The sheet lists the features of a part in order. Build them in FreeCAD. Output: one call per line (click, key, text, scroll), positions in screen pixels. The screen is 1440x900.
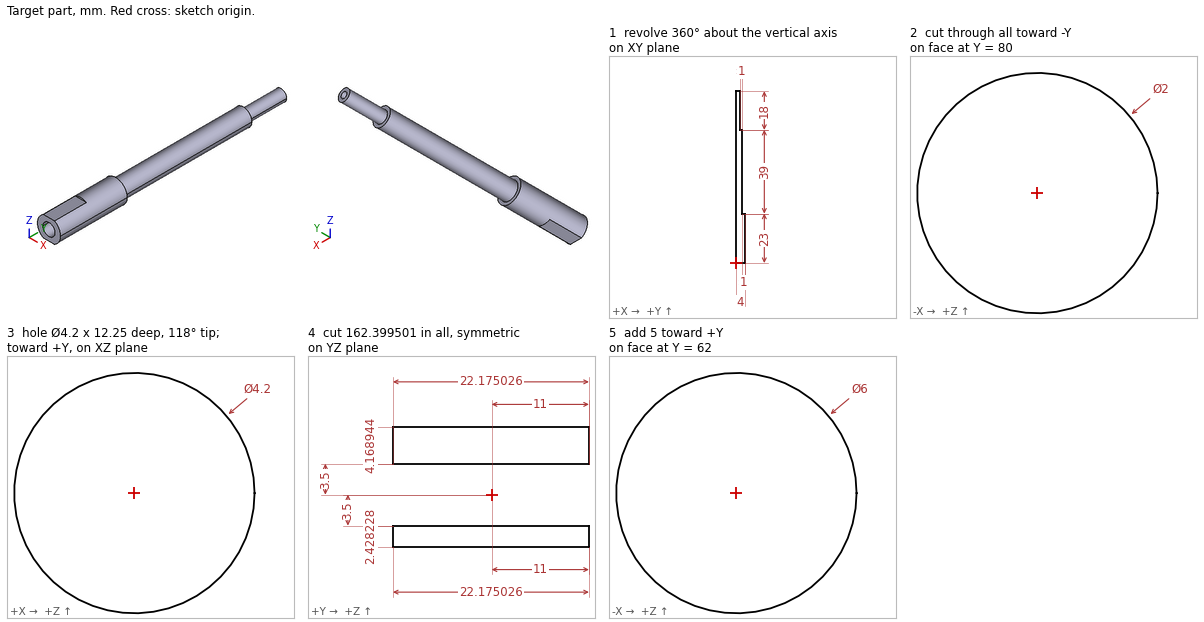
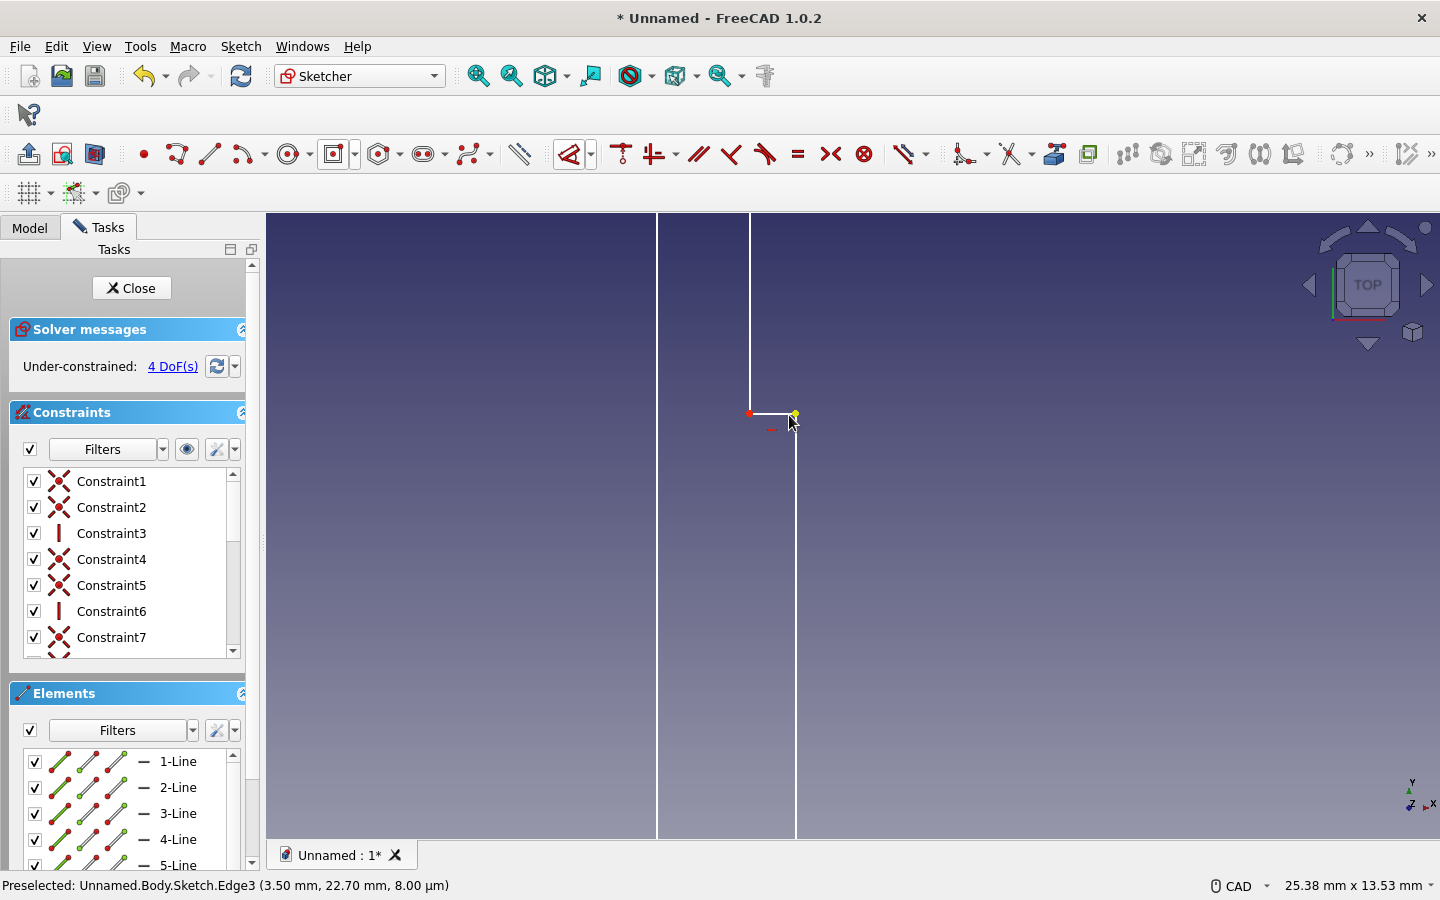
click(782, 414)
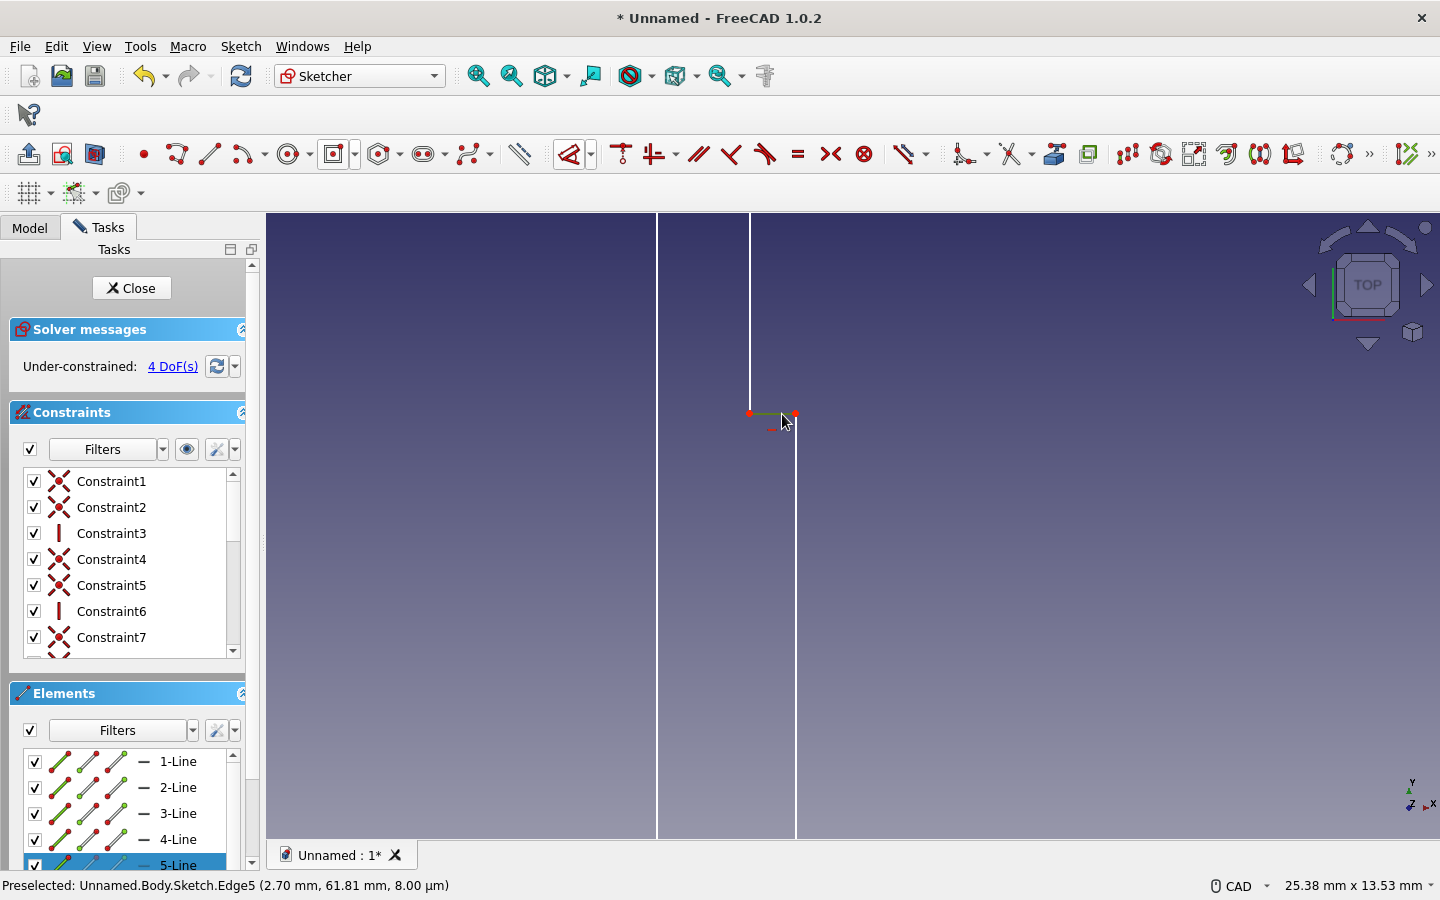
key(l)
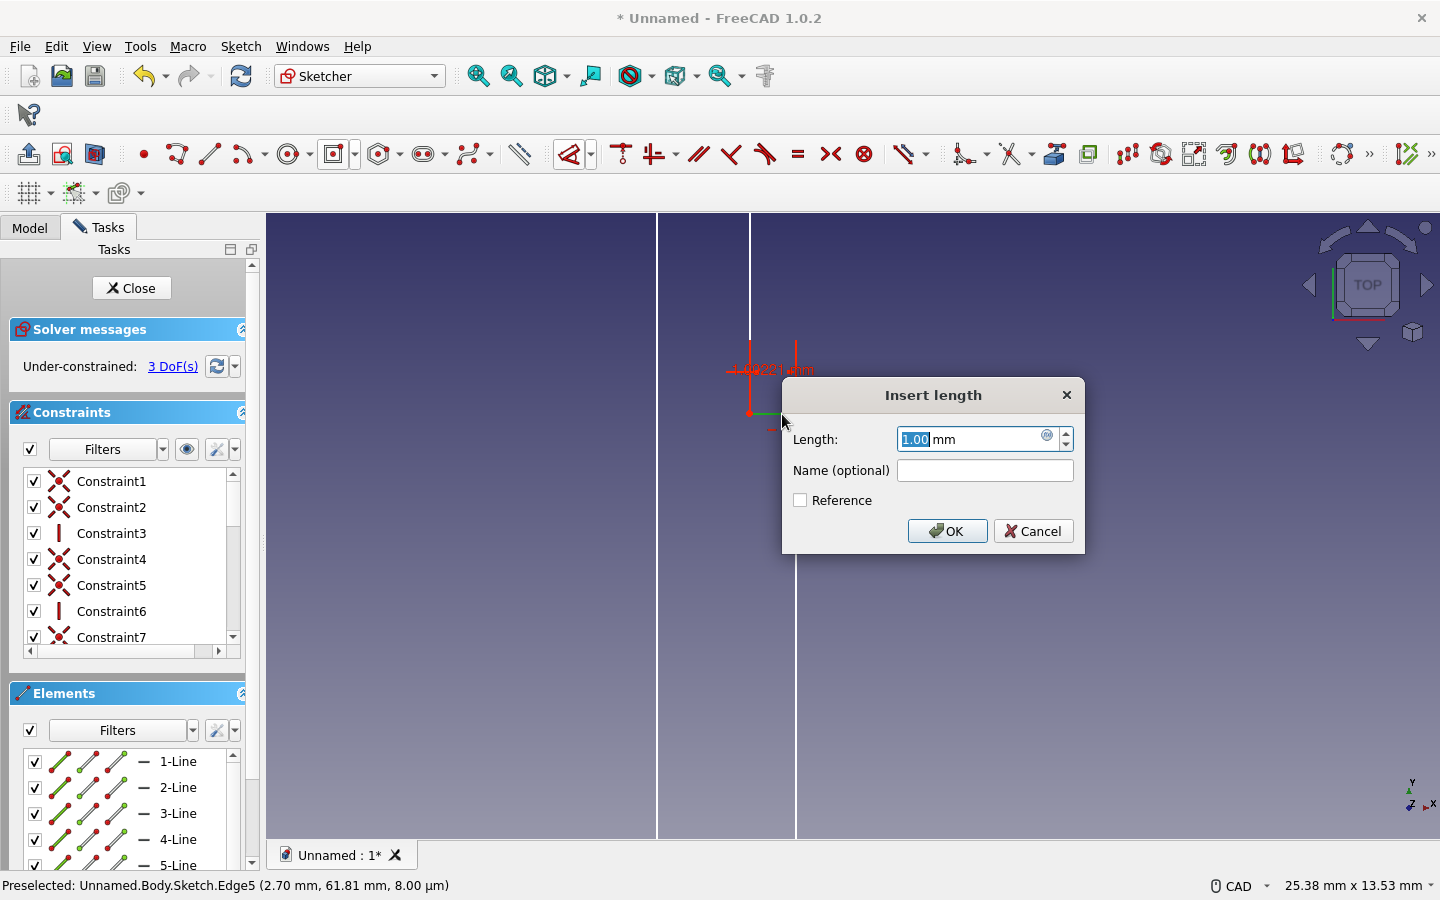
text(1)
key(Return)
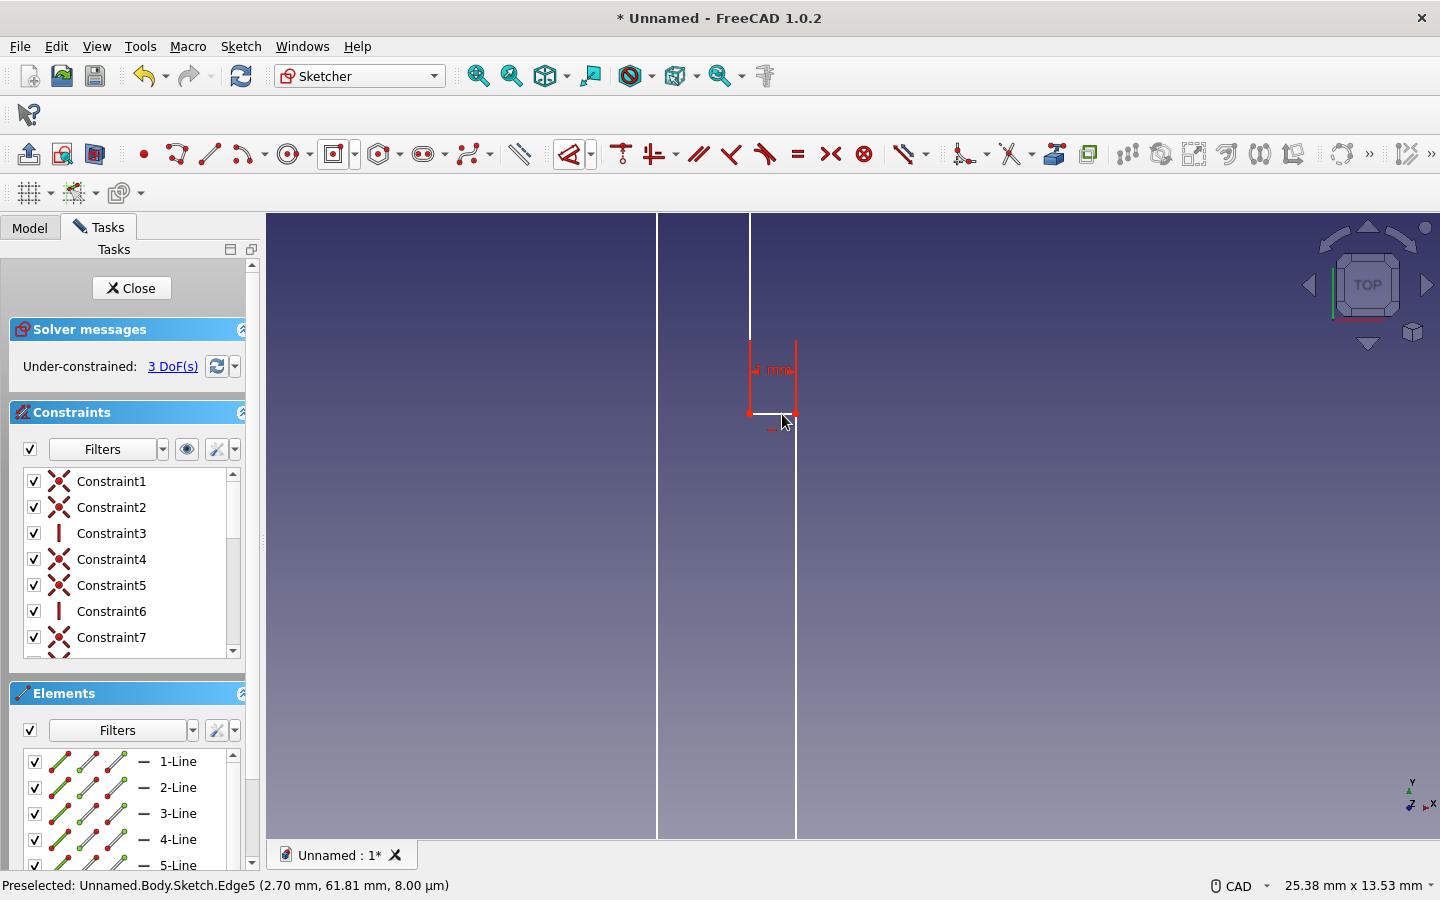
scroll(789, 414, down, 11)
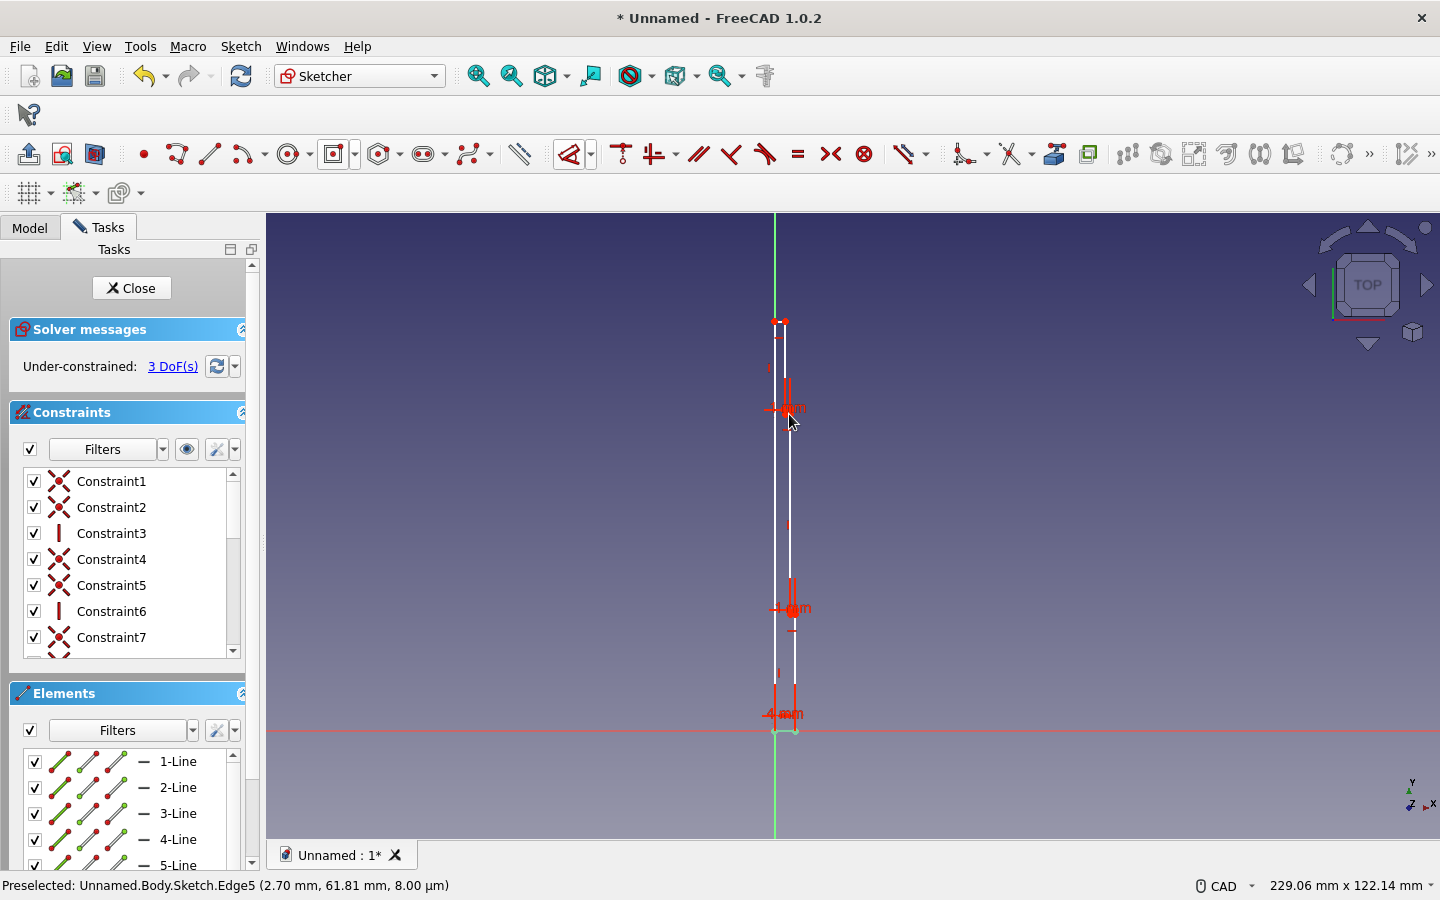
click(795, 696)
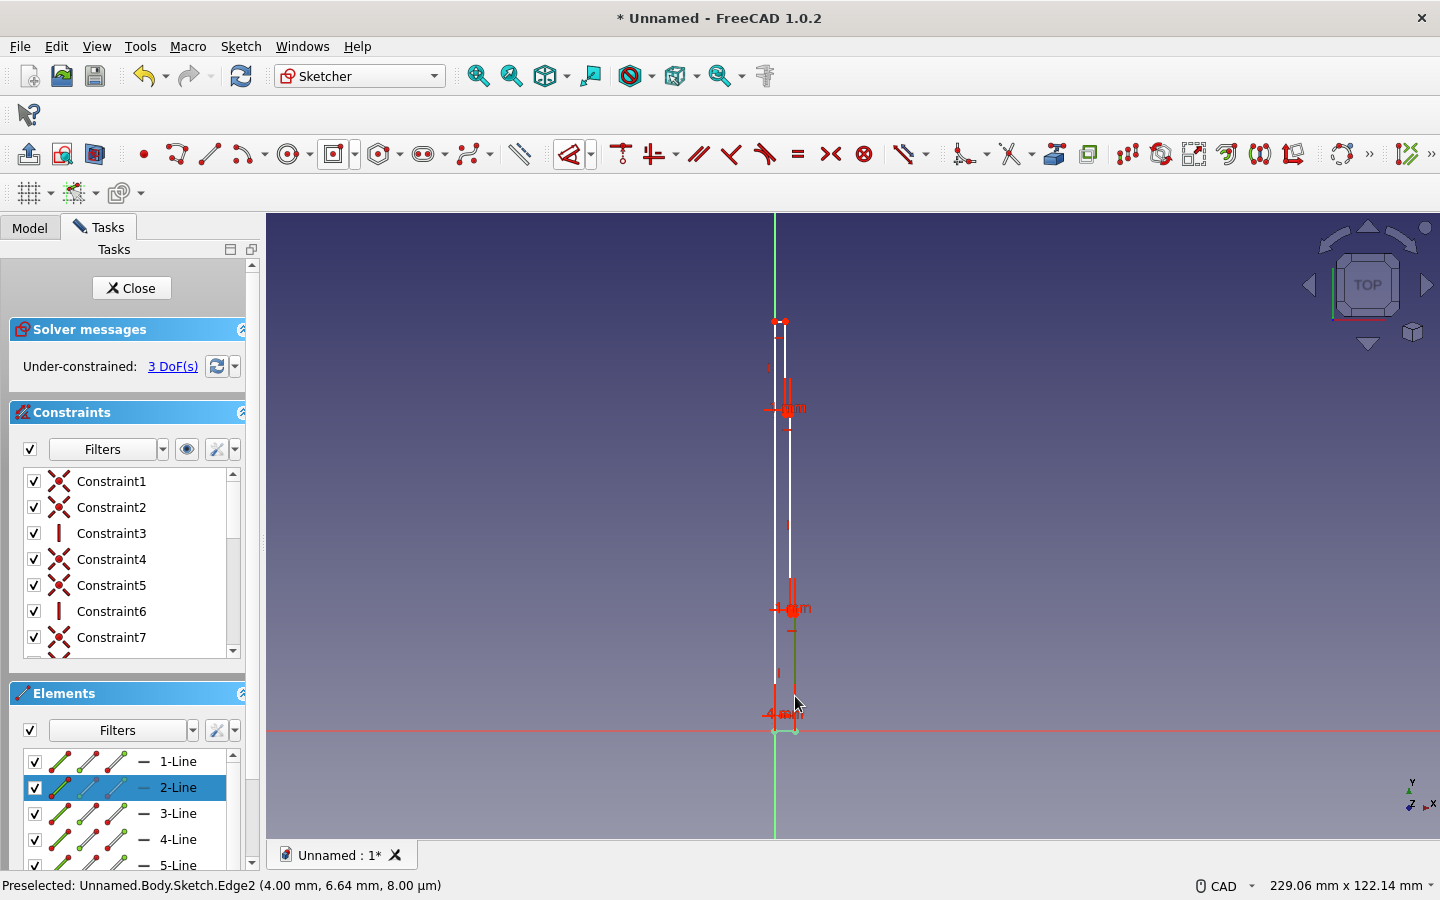
key(i)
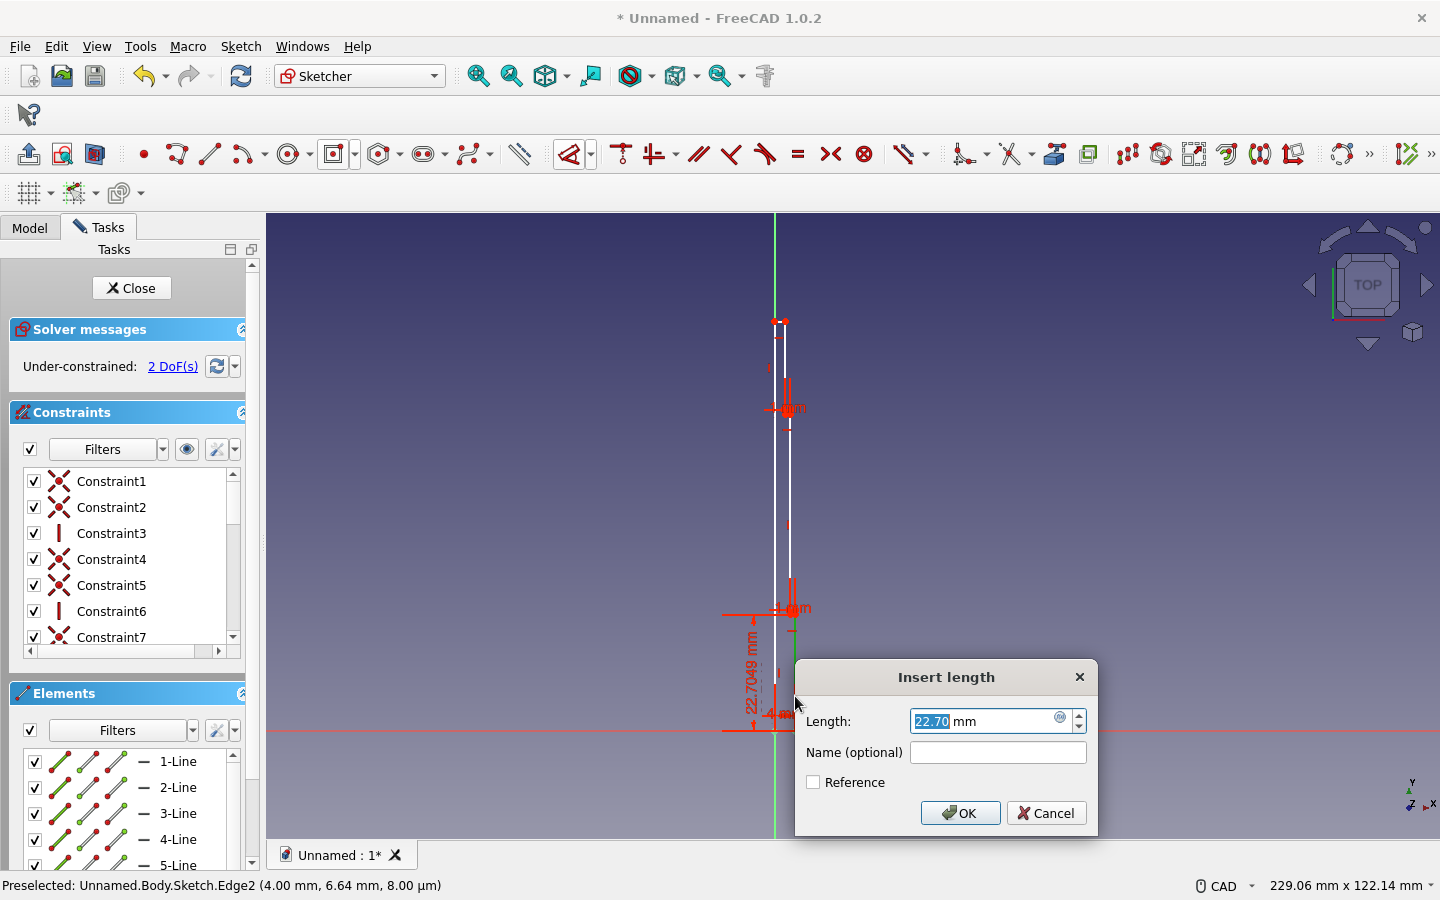
text(23)
key(Return)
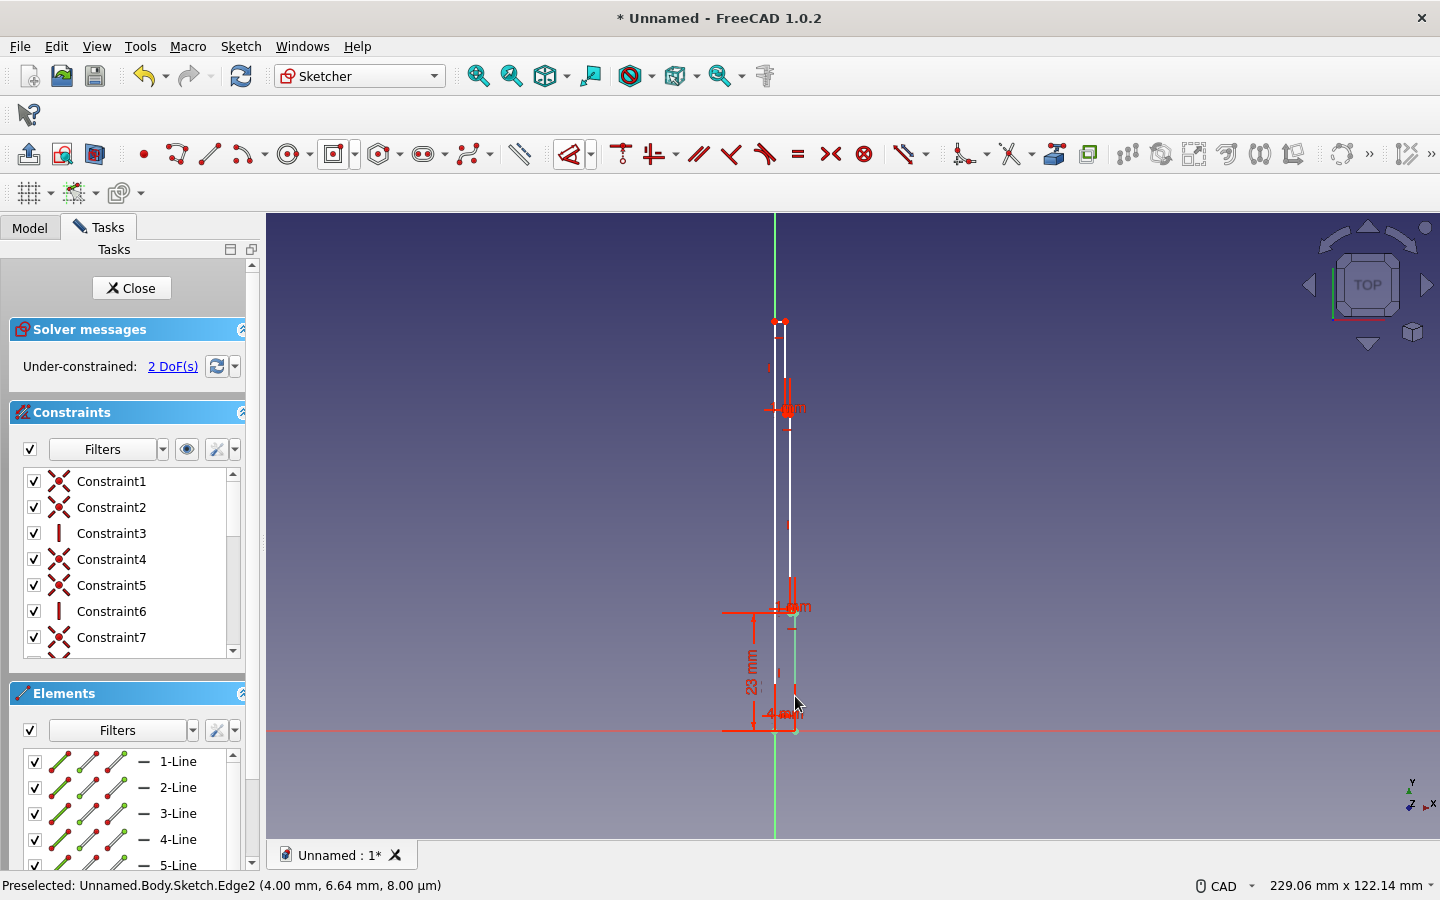
click(790, 553)